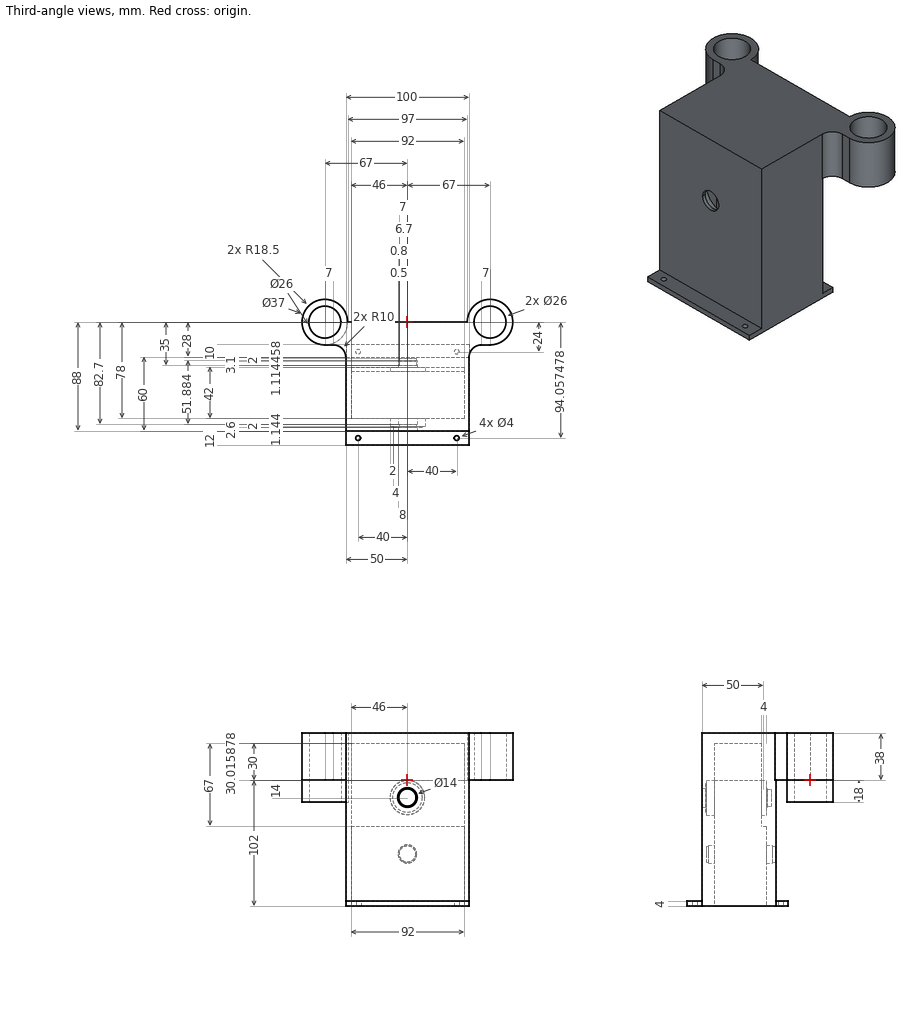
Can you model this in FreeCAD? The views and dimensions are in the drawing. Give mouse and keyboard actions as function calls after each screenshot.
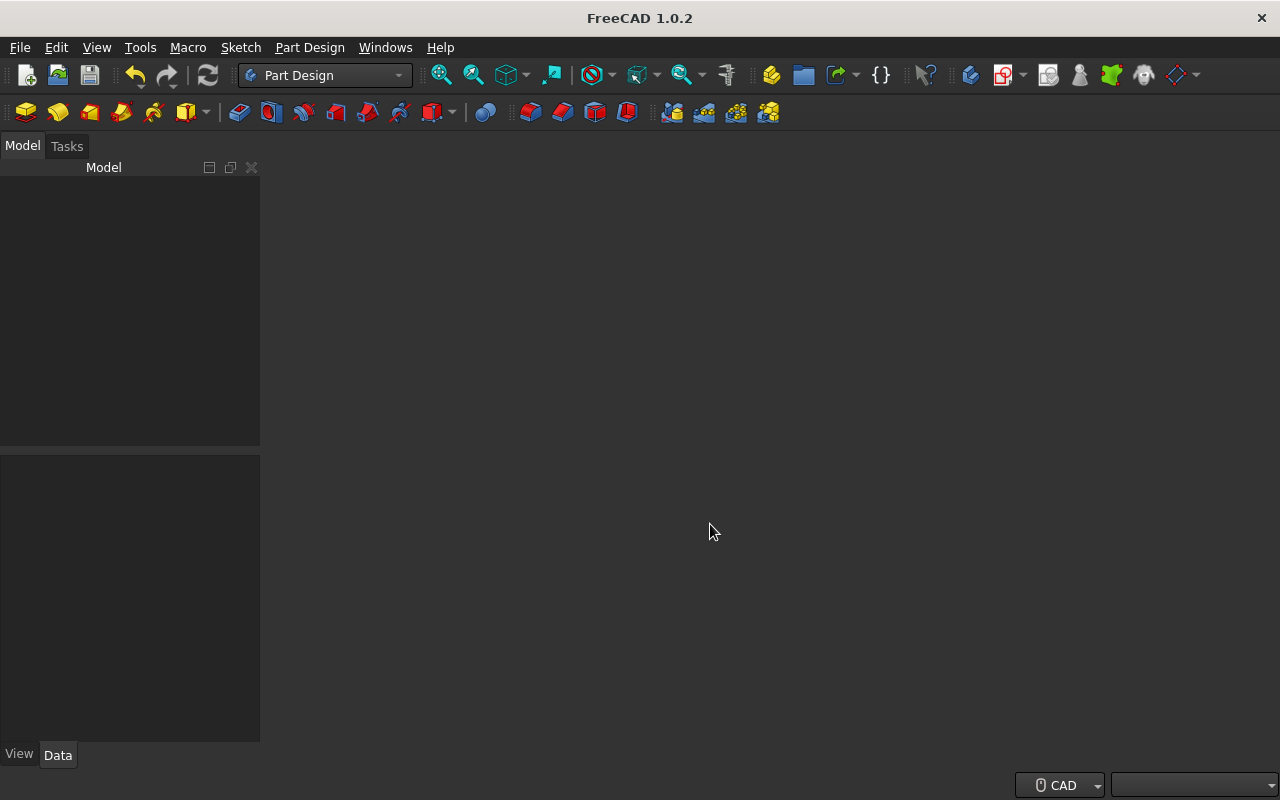
key(ctrl+n)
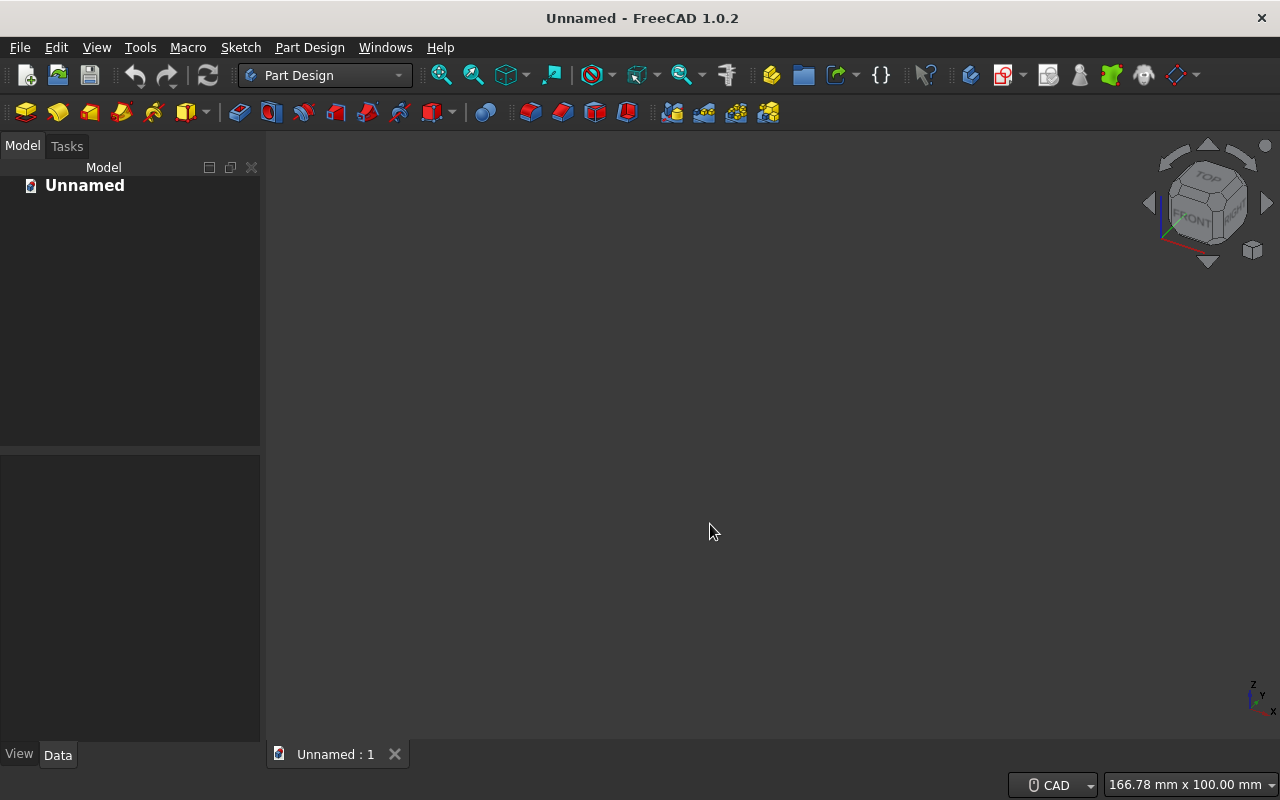
click(1004, 76)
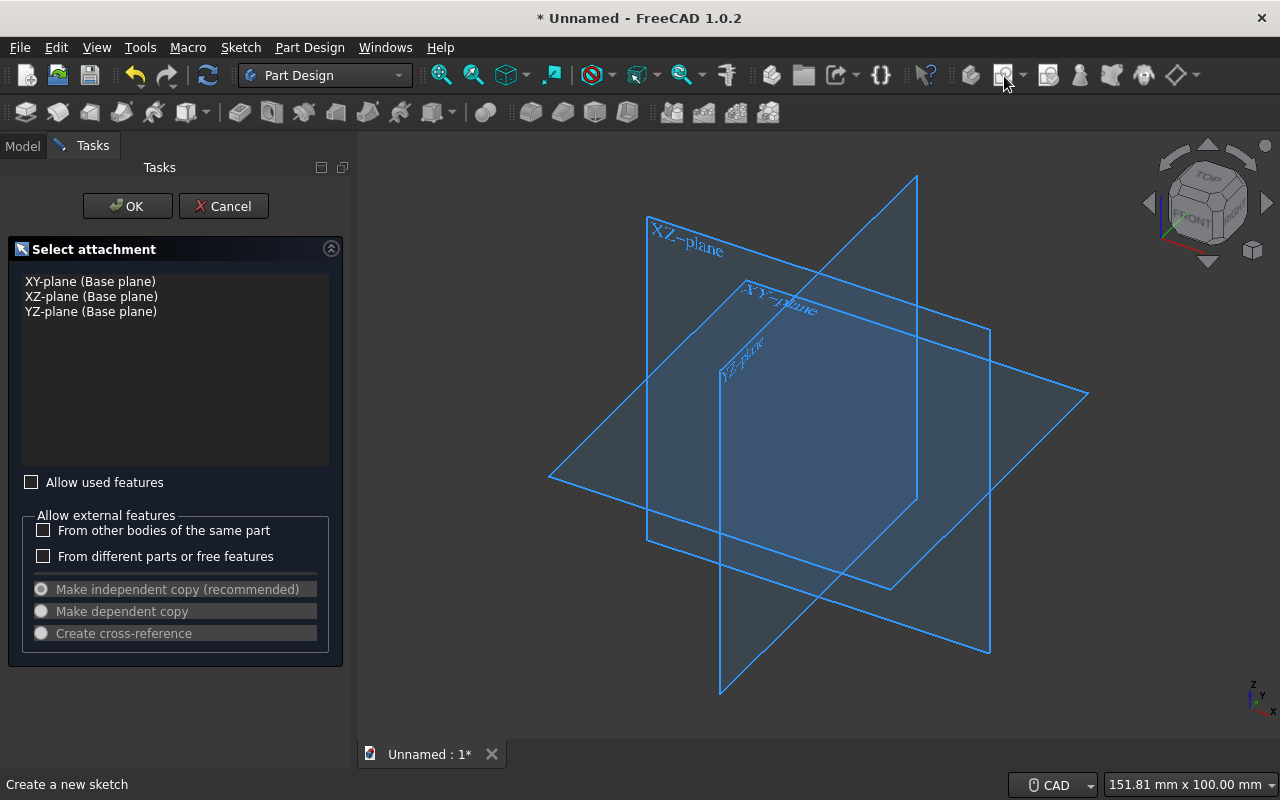
click(82, 282)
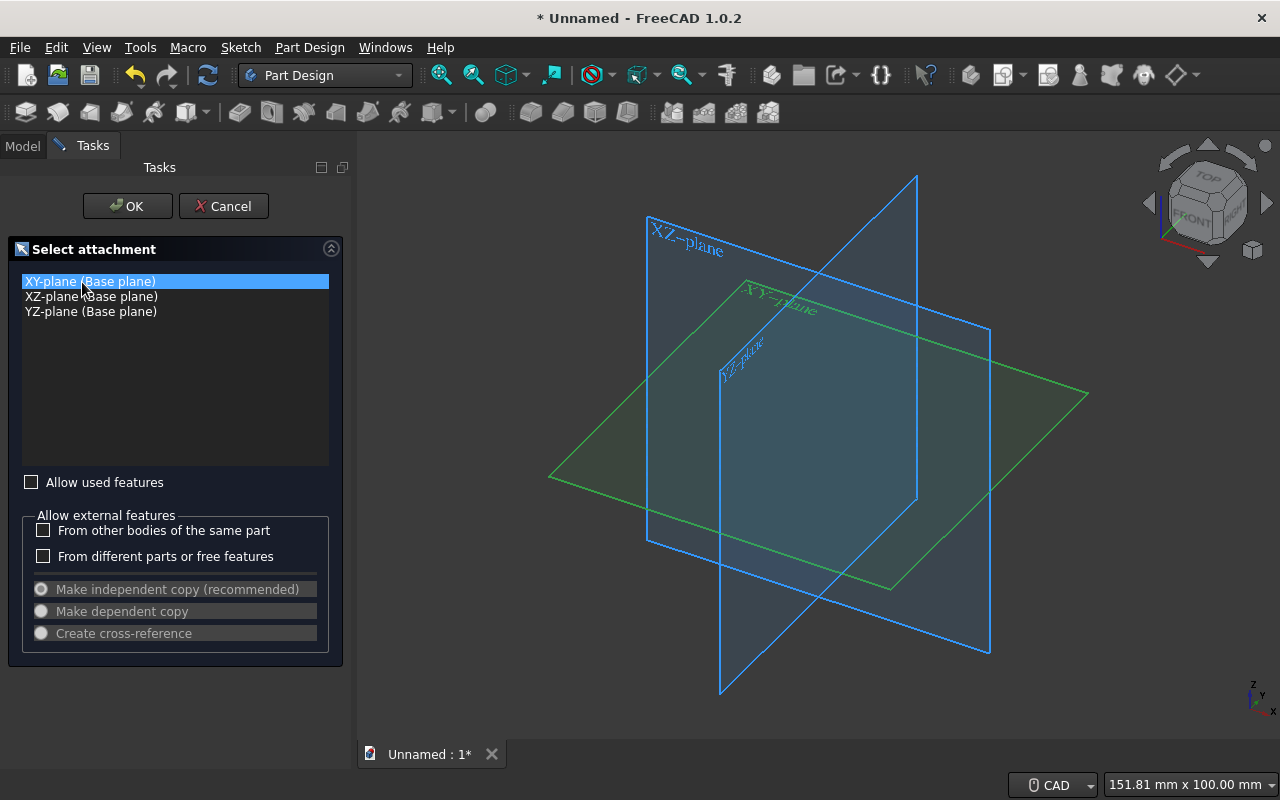
click(128, 206)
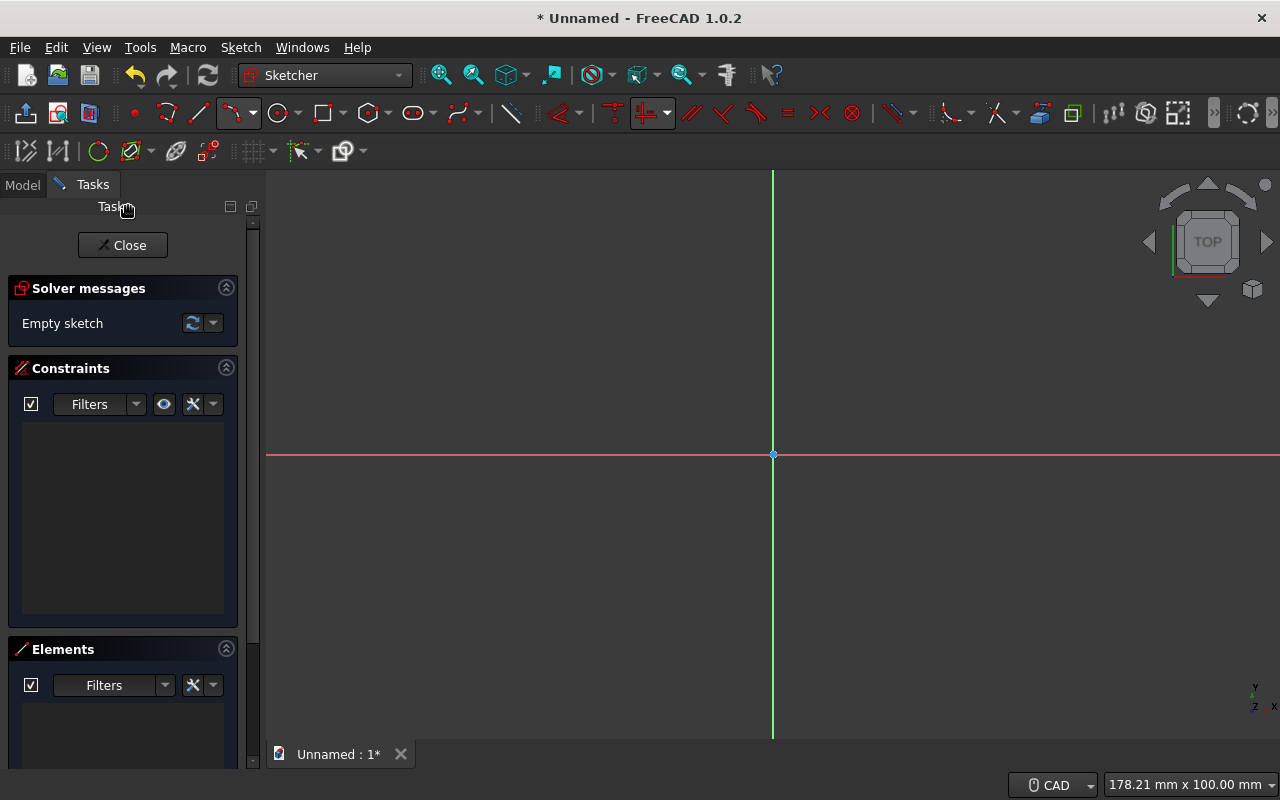
scroll(621, 198, down, 3)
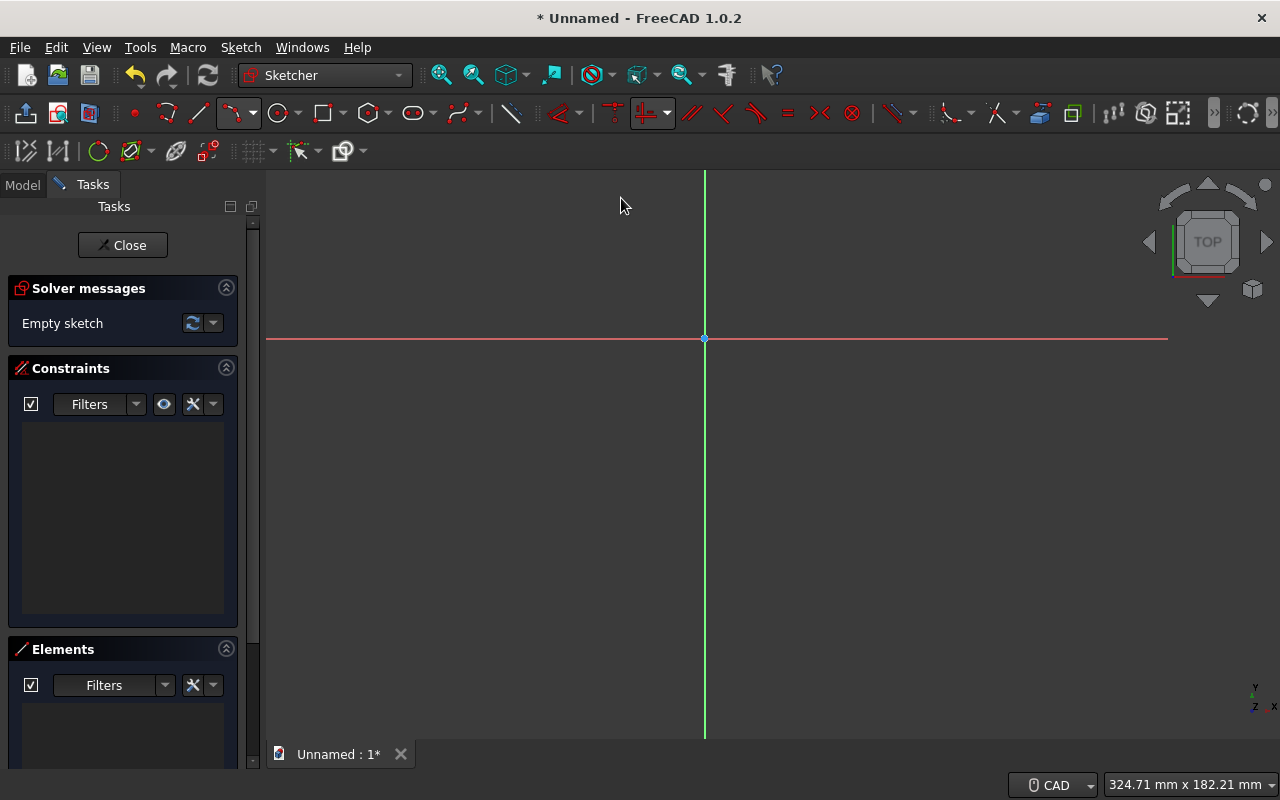
key(g)
key(l)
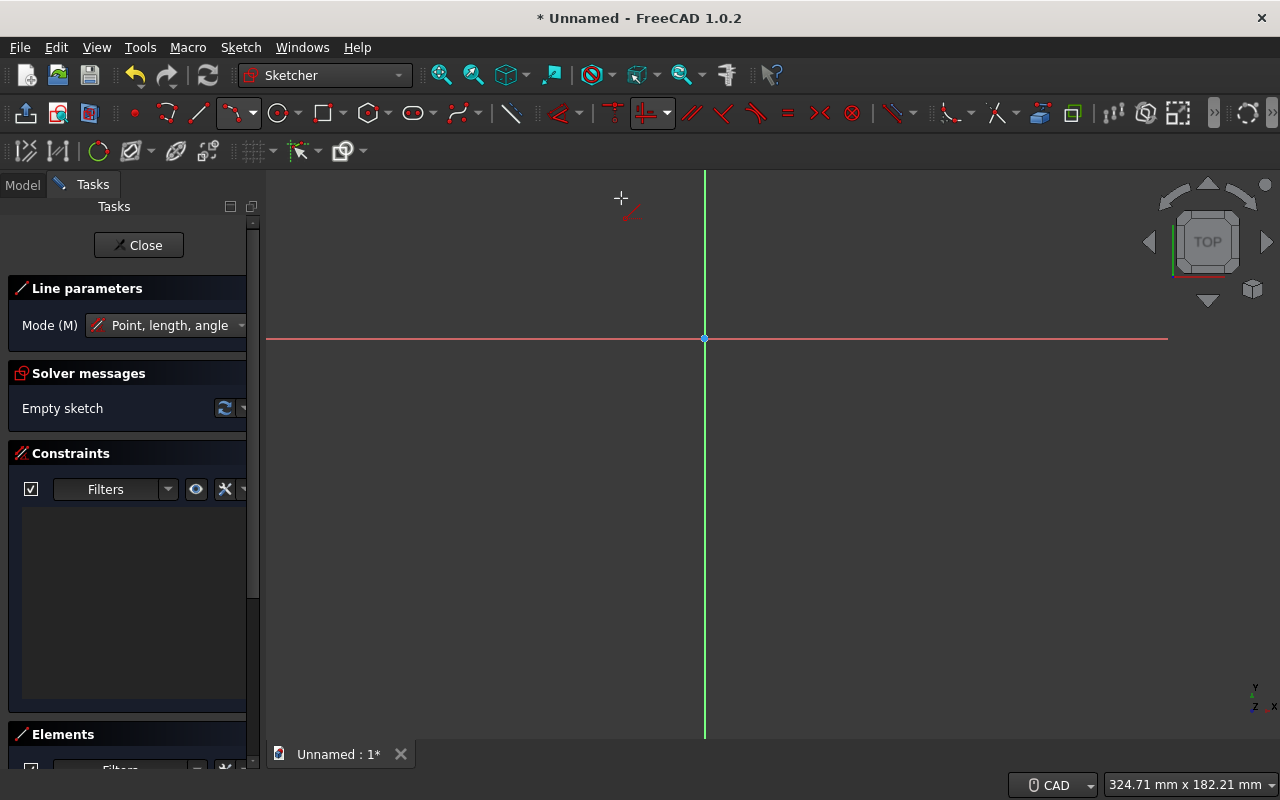
click(856, 339)
click(553, 348)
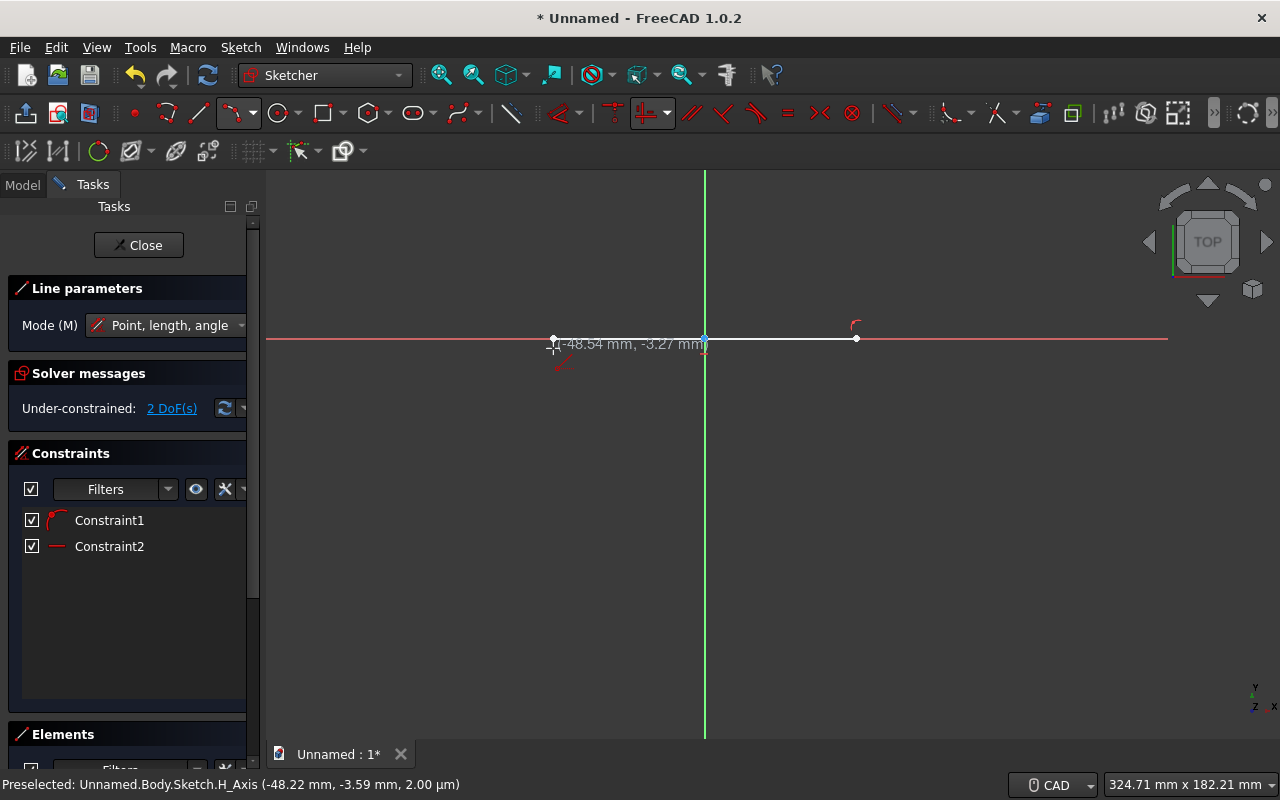
click(495, 397)
click(517, 397)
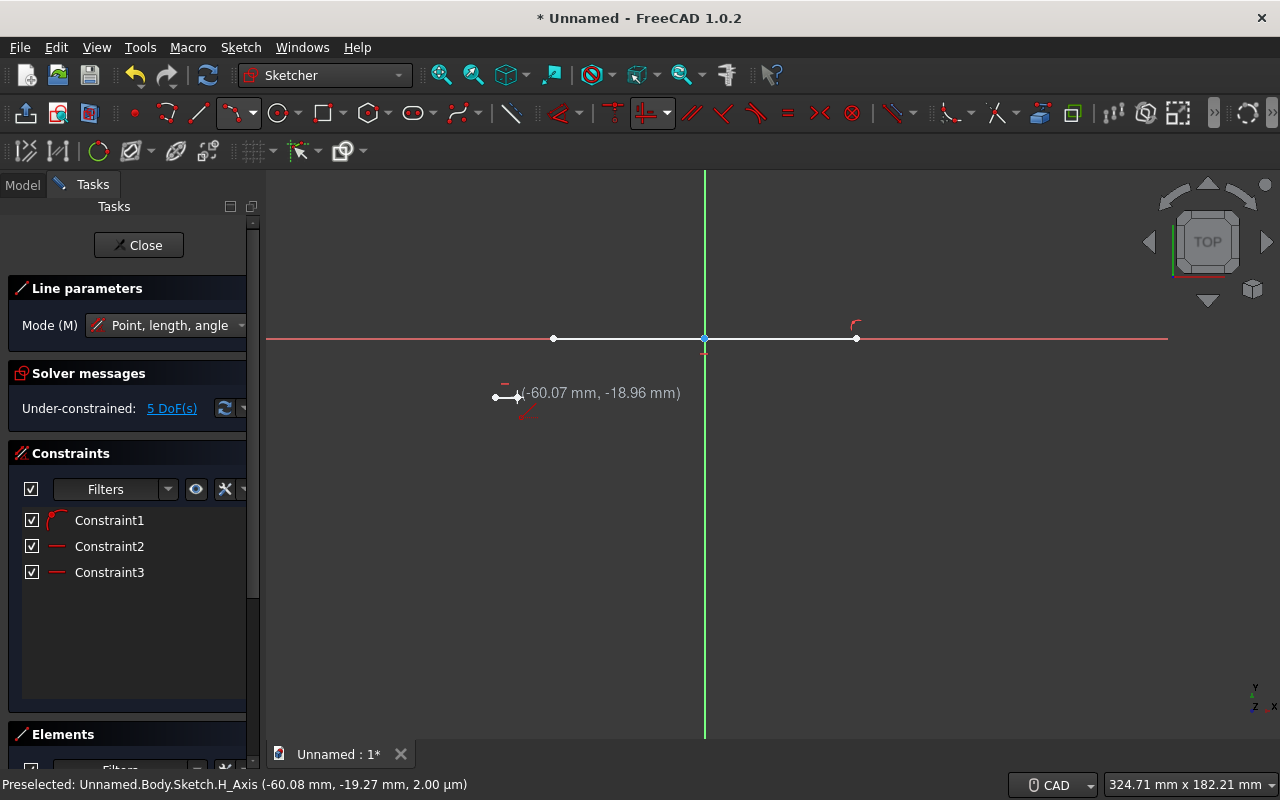
key(g)
key(m)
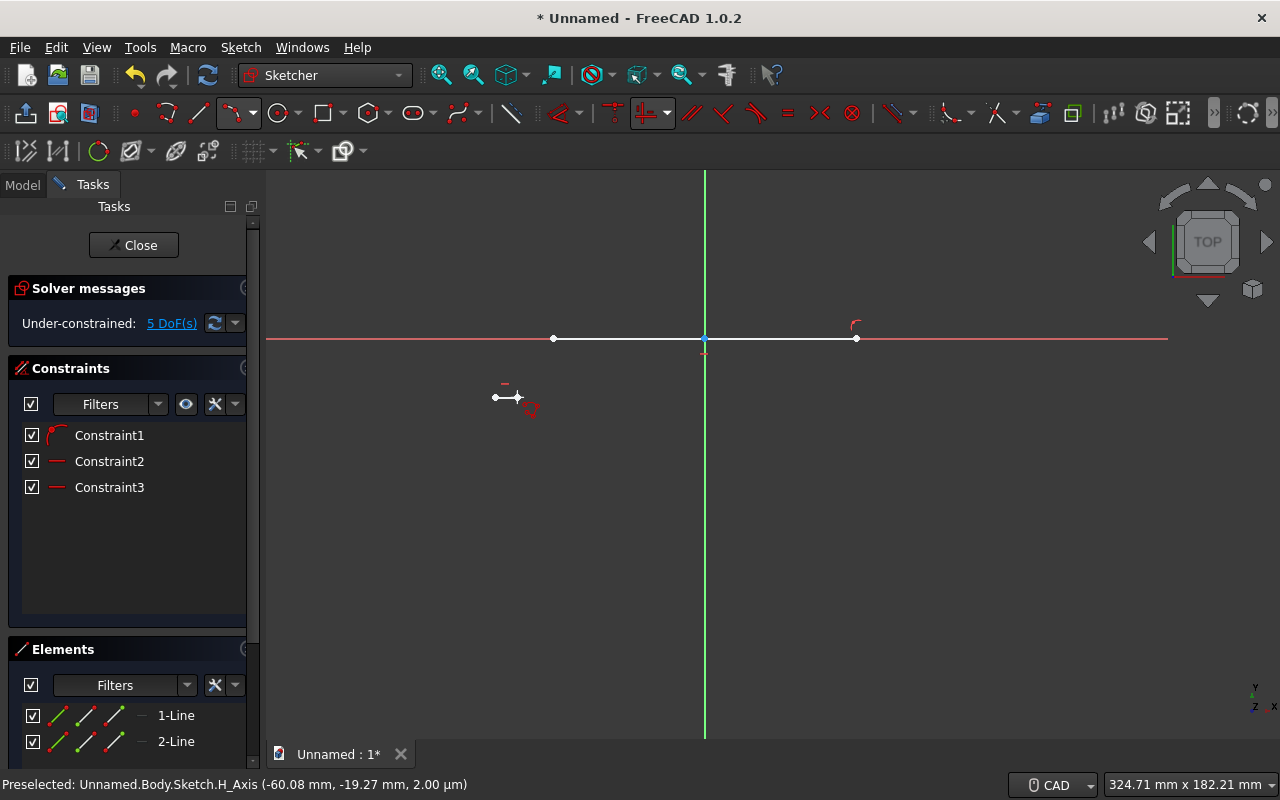
click(548, 428)
click(548, 614)
click(861, 614)
click(861, 428)
right_click(861, 428)